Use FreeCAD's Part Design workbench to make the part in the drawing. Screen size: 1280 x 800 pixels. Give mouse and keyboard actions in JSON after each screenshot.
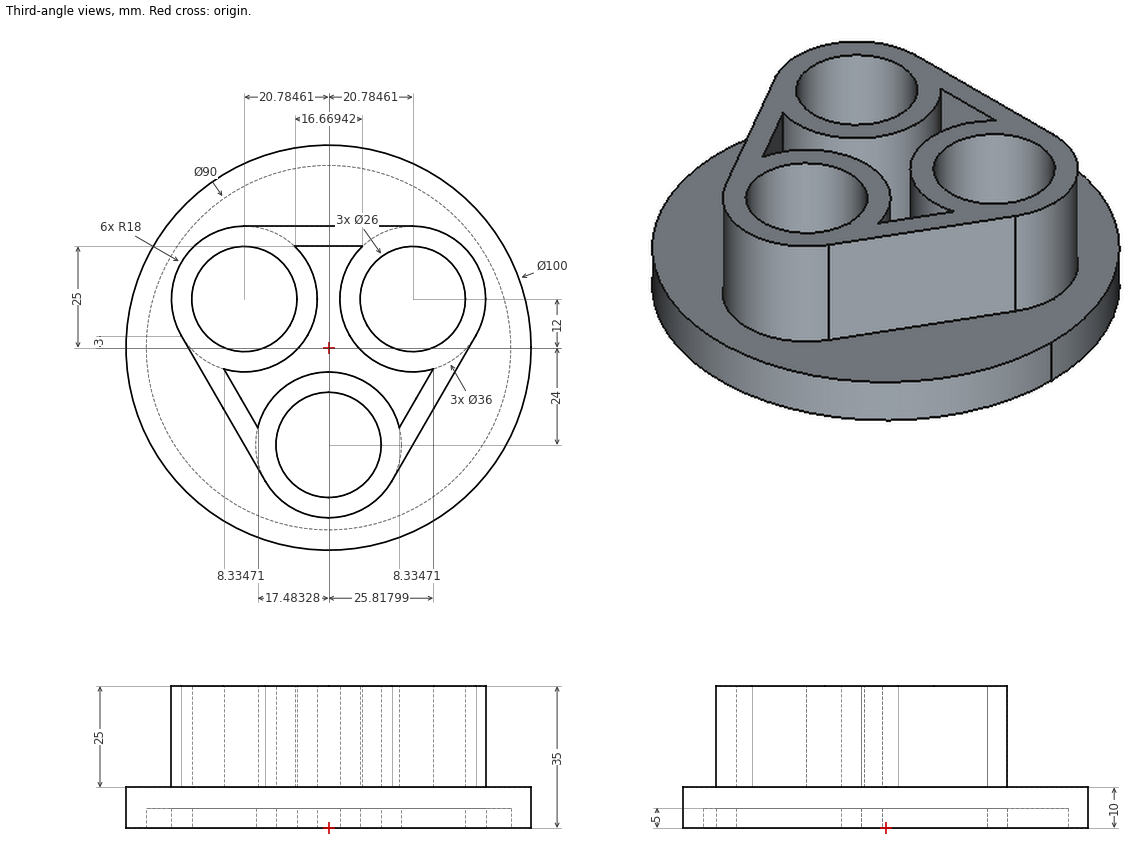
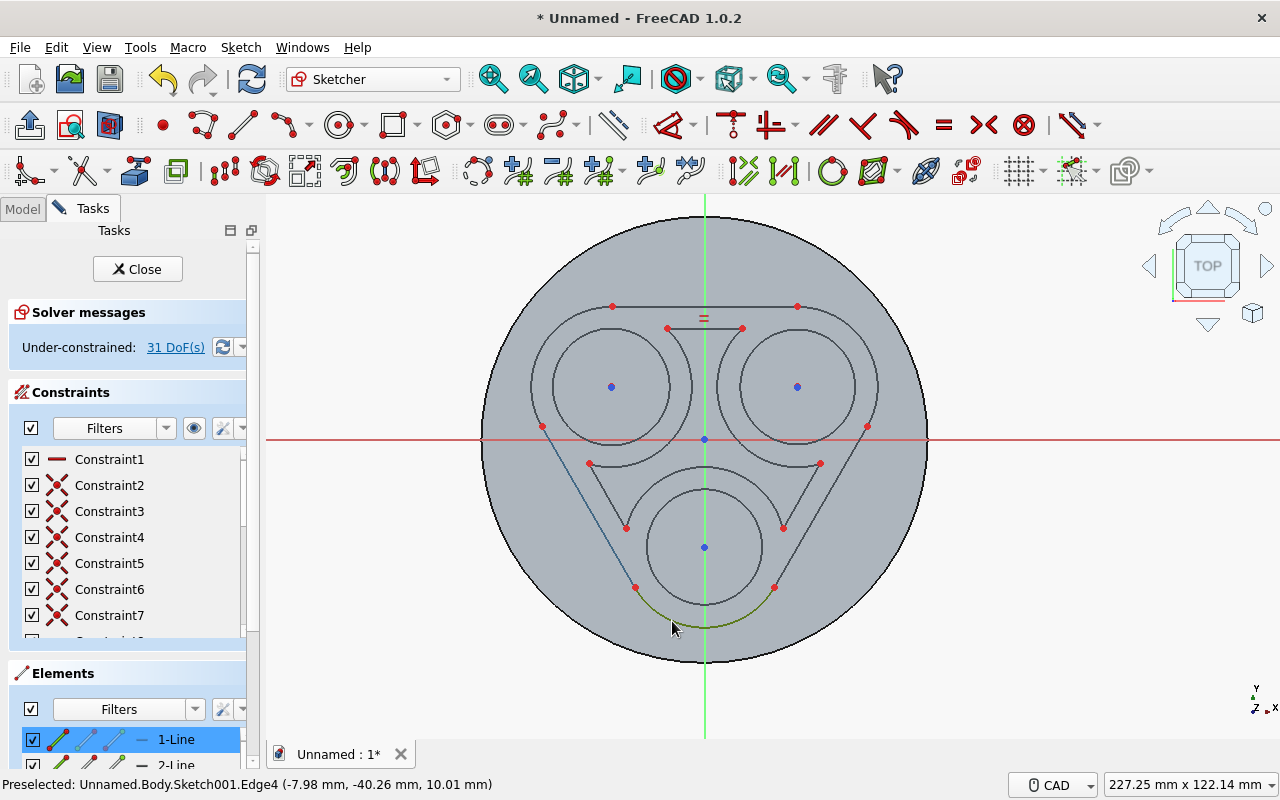
{"action": "left_click", "coordinate": [904, 126]}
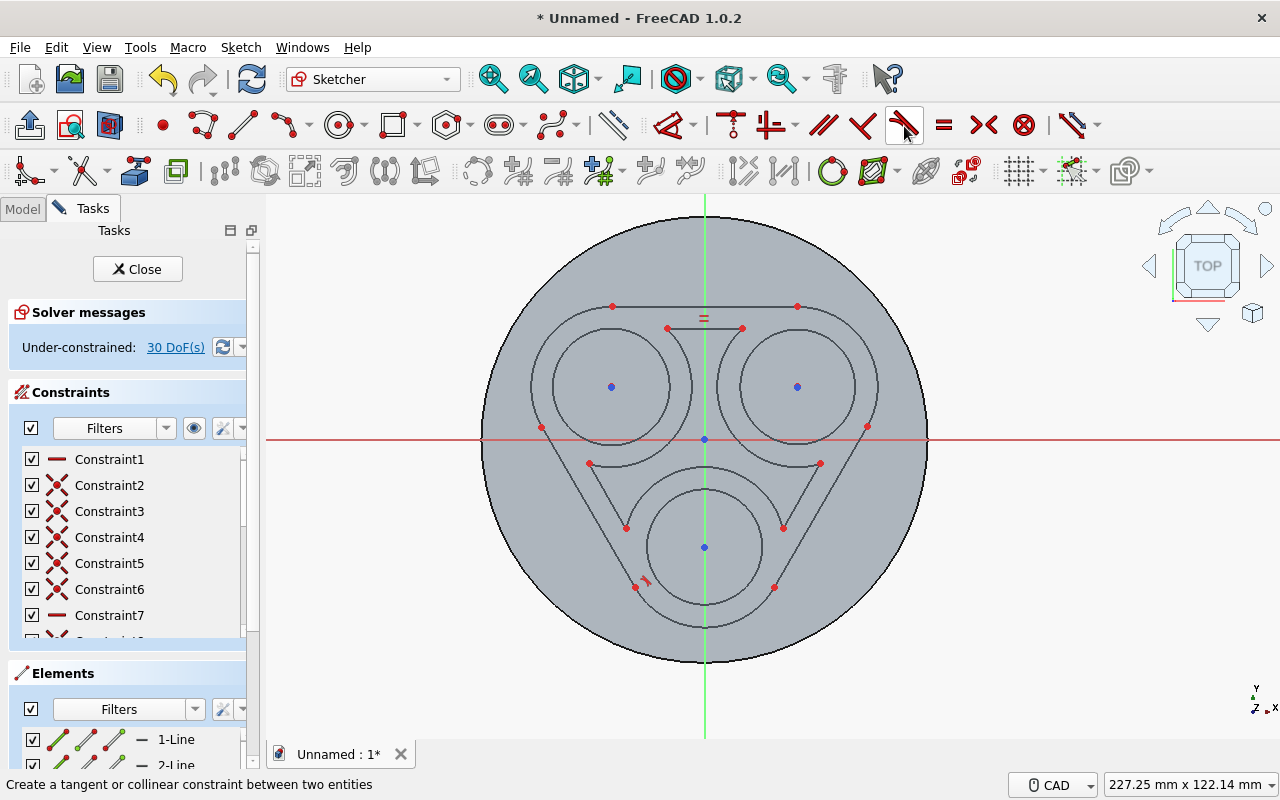
{"action": "left_click", "coordinate": [570, 475]}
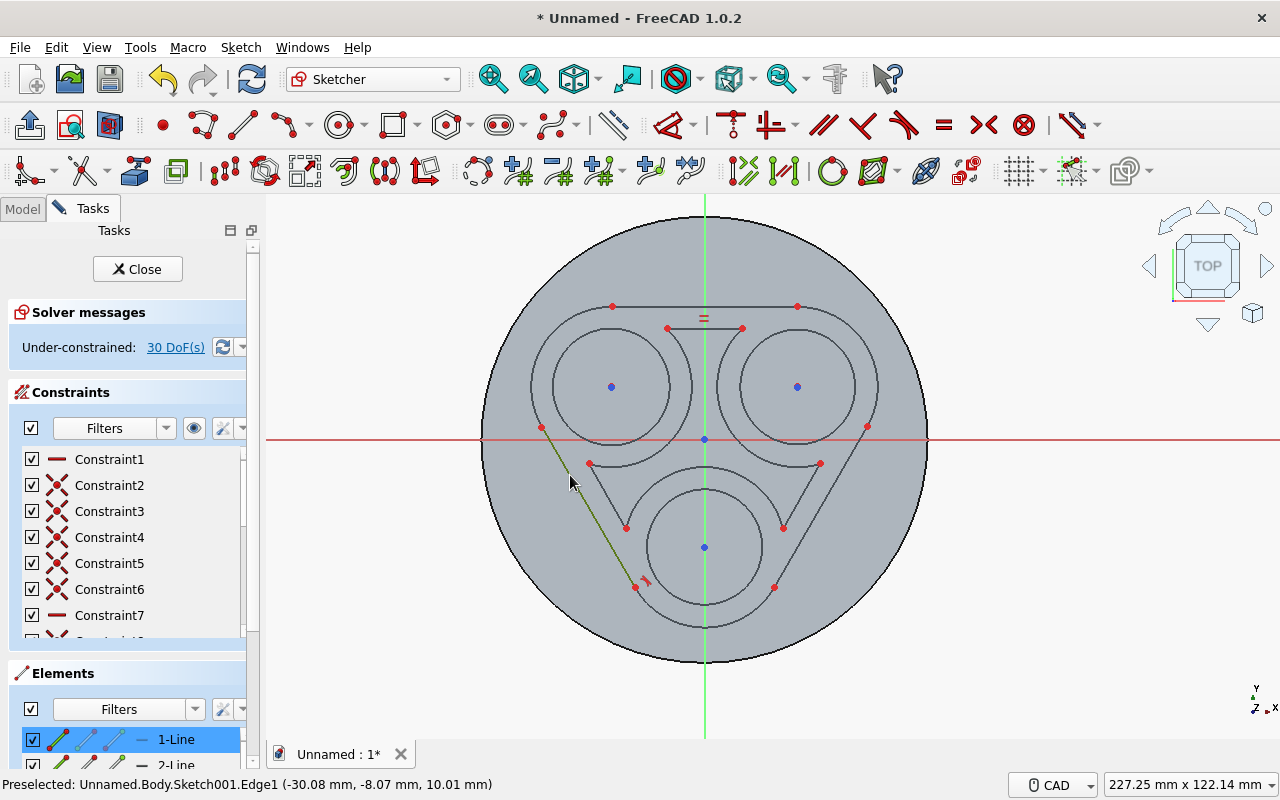
{"action": "left_click", "coordinate": [565, 322]}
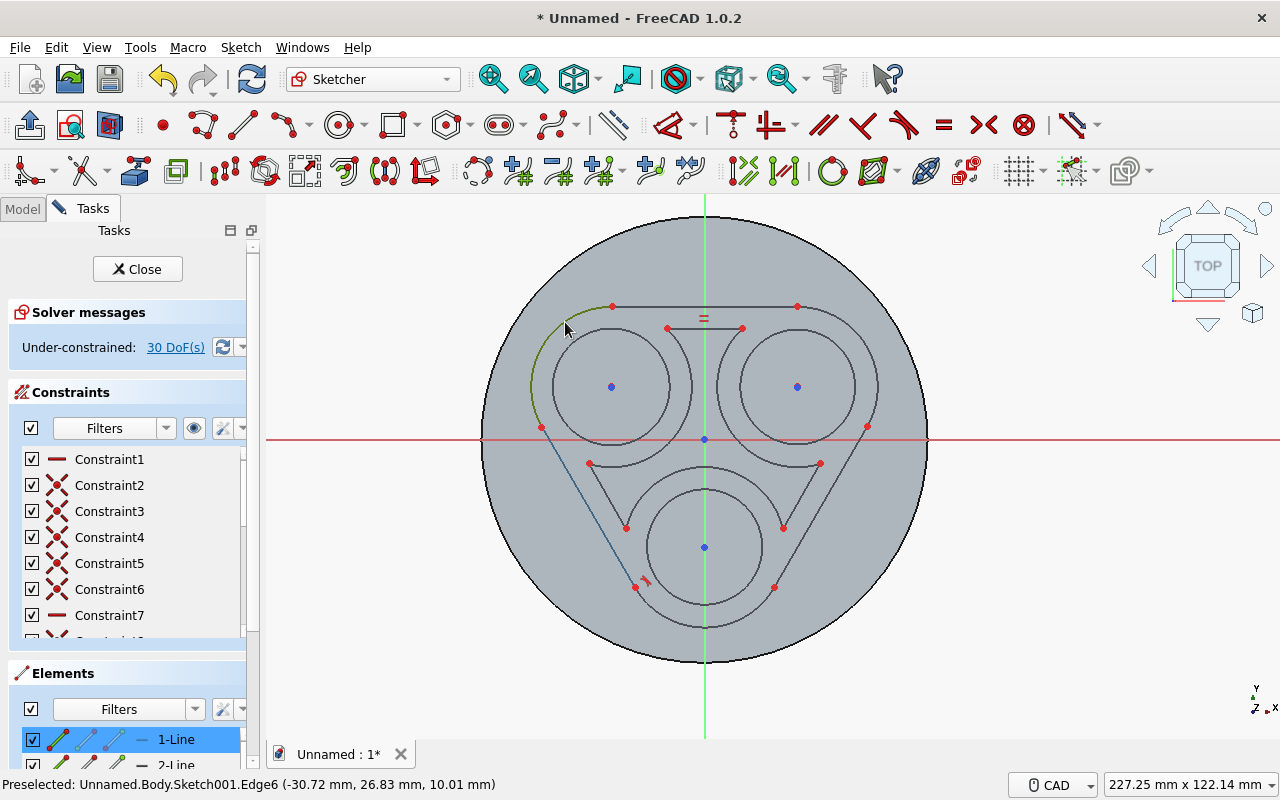
{"action": "left_click", "coordinate": [904, 126]}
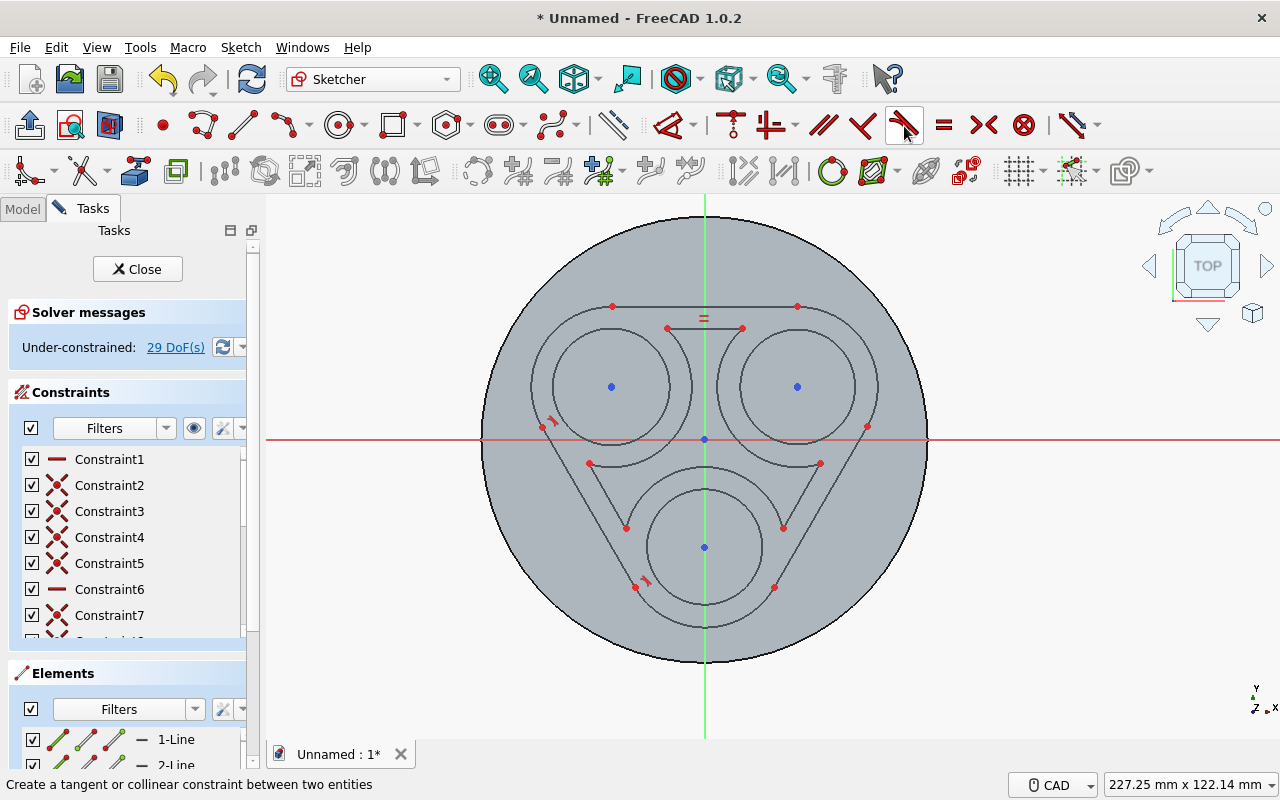
{"action": "left_click", "coordinate": [802, 540]}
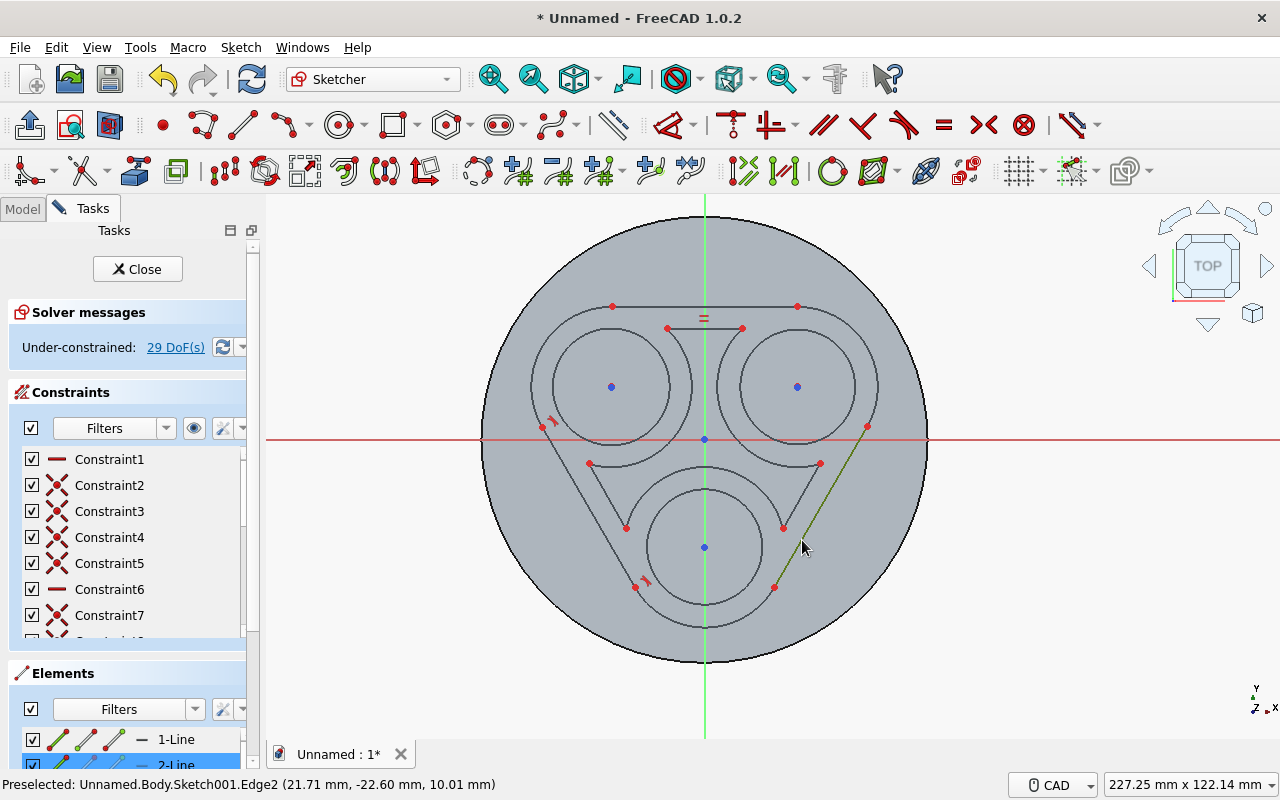
{"action": "left_click", "coordinate": [672, 621]}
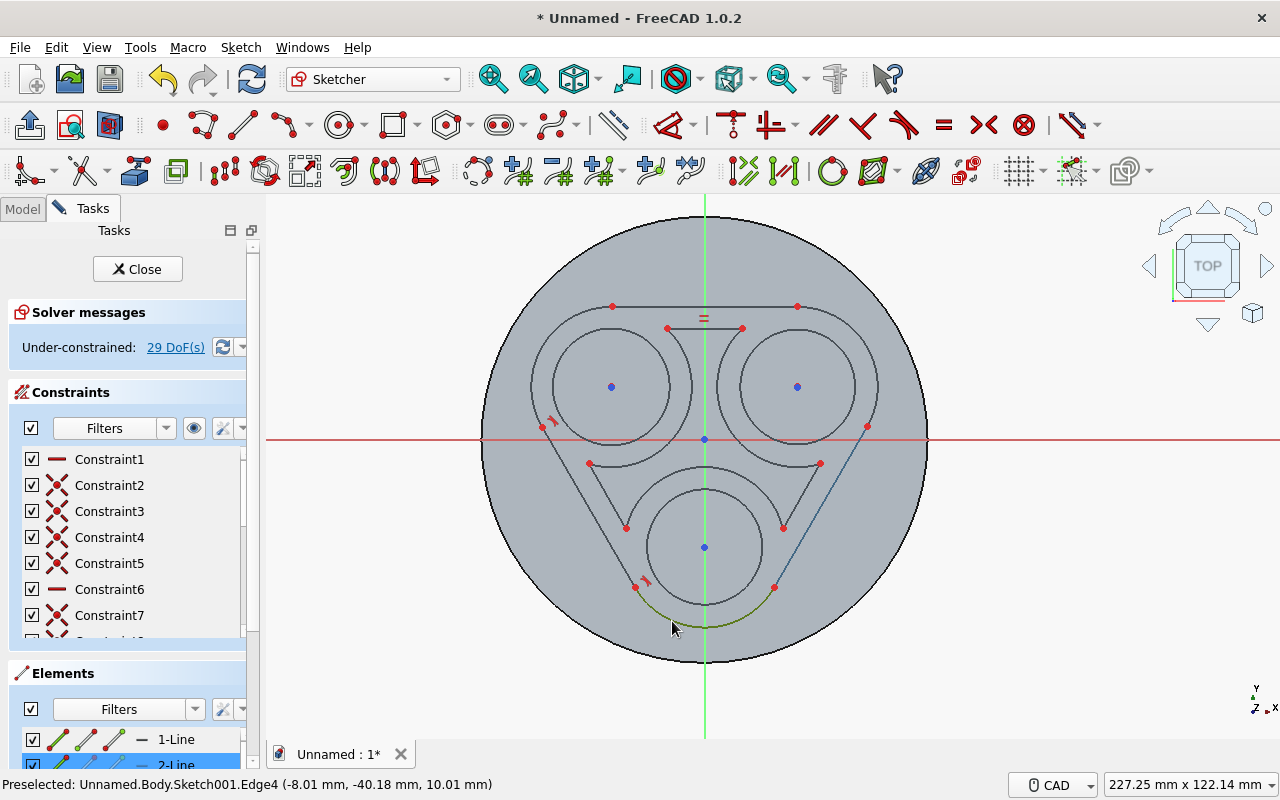
{"action": "left_click", "coordinate": [904, 126]}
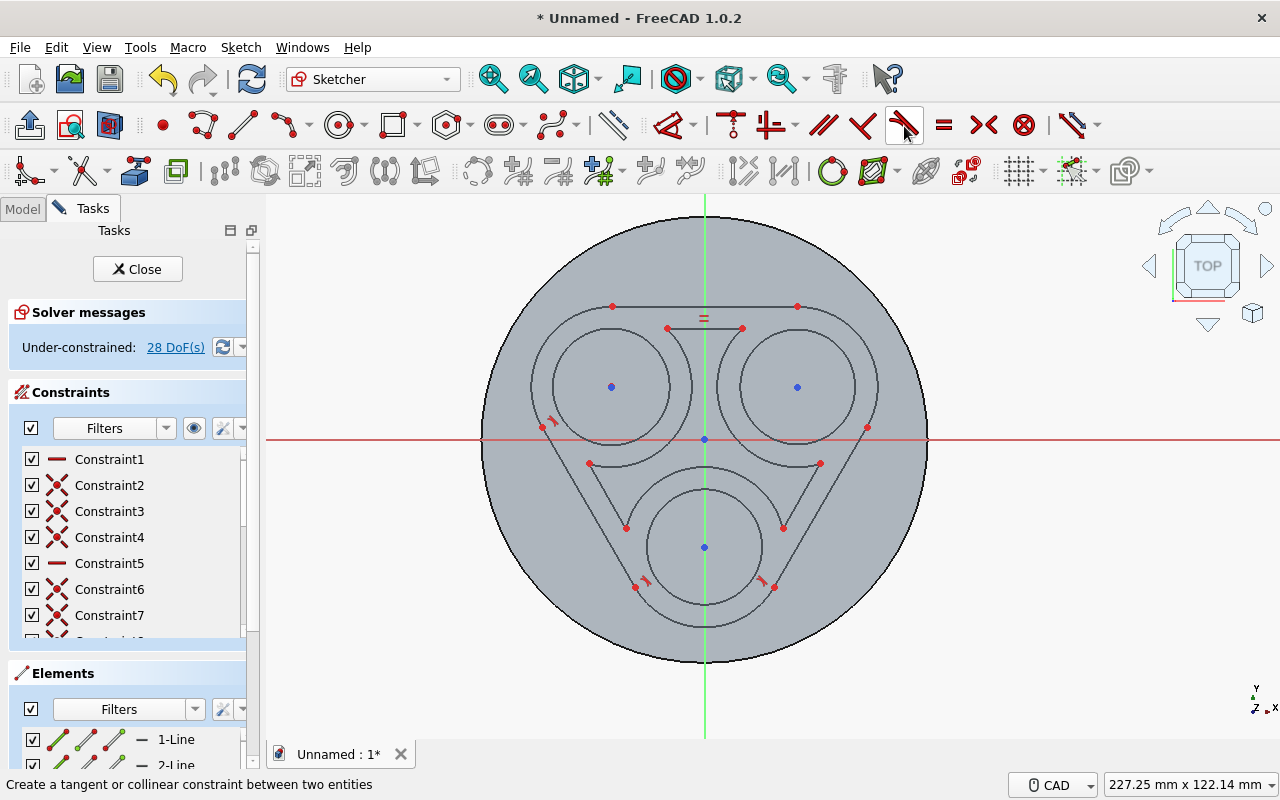
{"action": "left_click", "coordinate": [802, 539]}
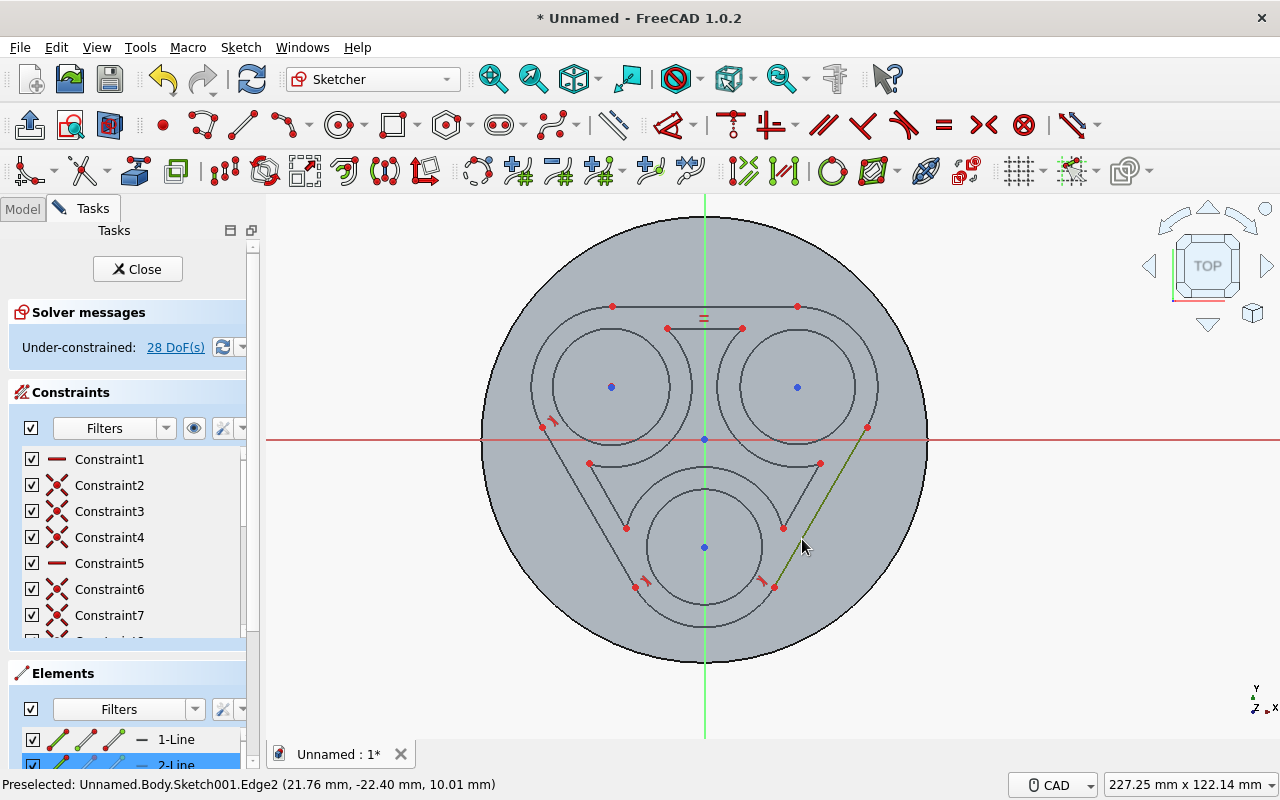
{"action": "left_click", "coordinate": [877, 378]}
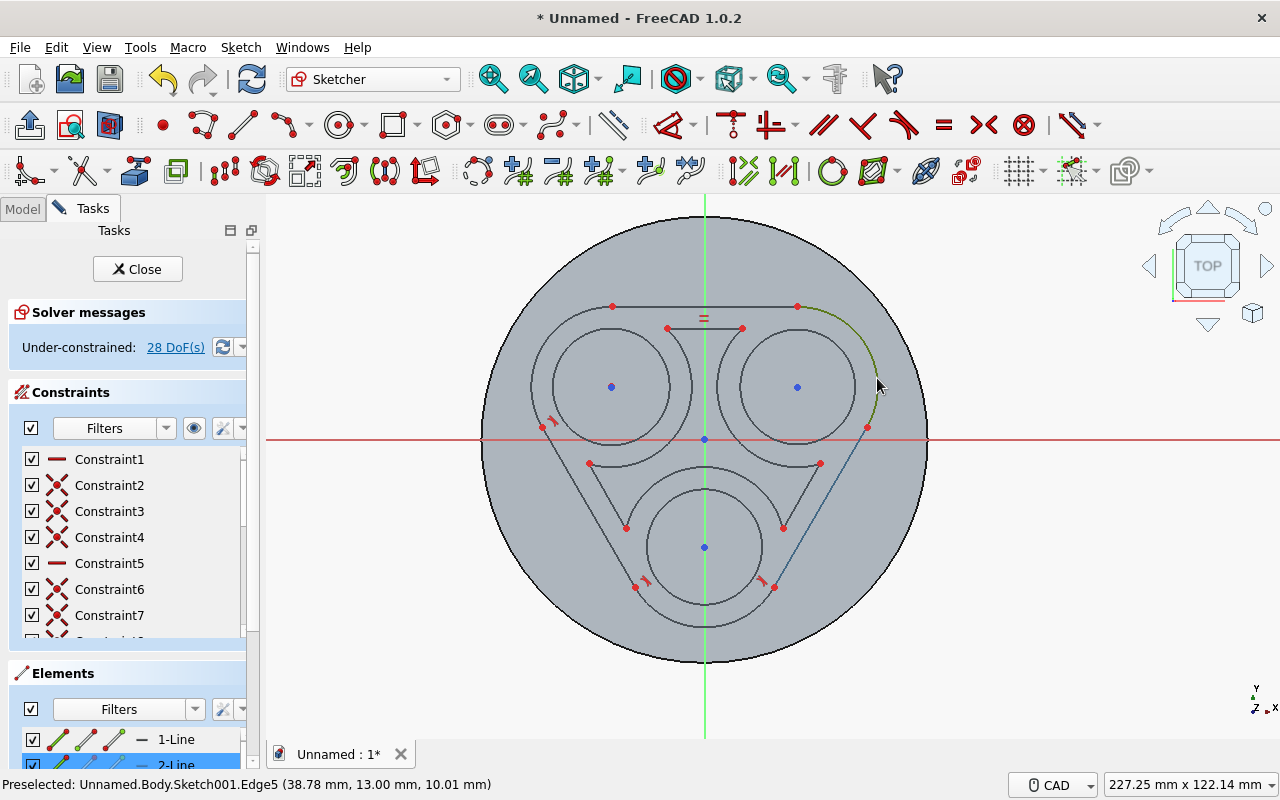
{"action": "key", "text": "t"}